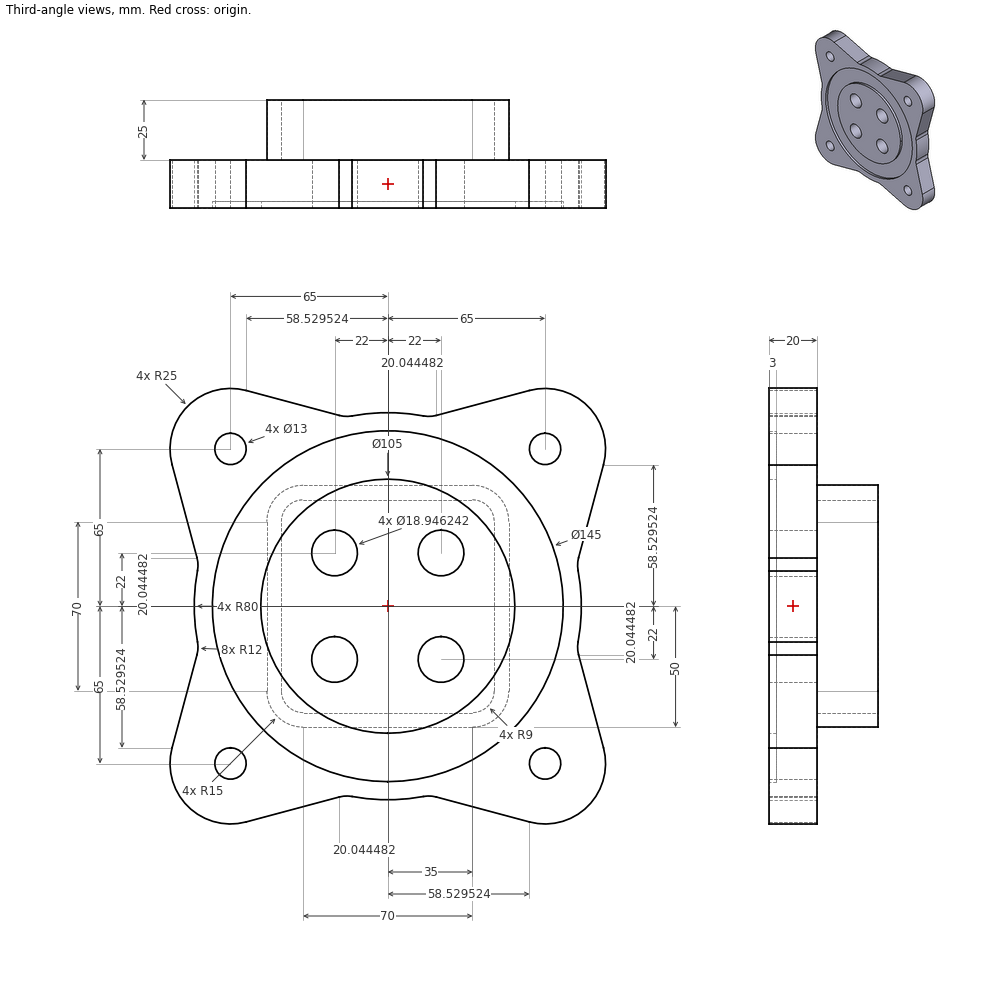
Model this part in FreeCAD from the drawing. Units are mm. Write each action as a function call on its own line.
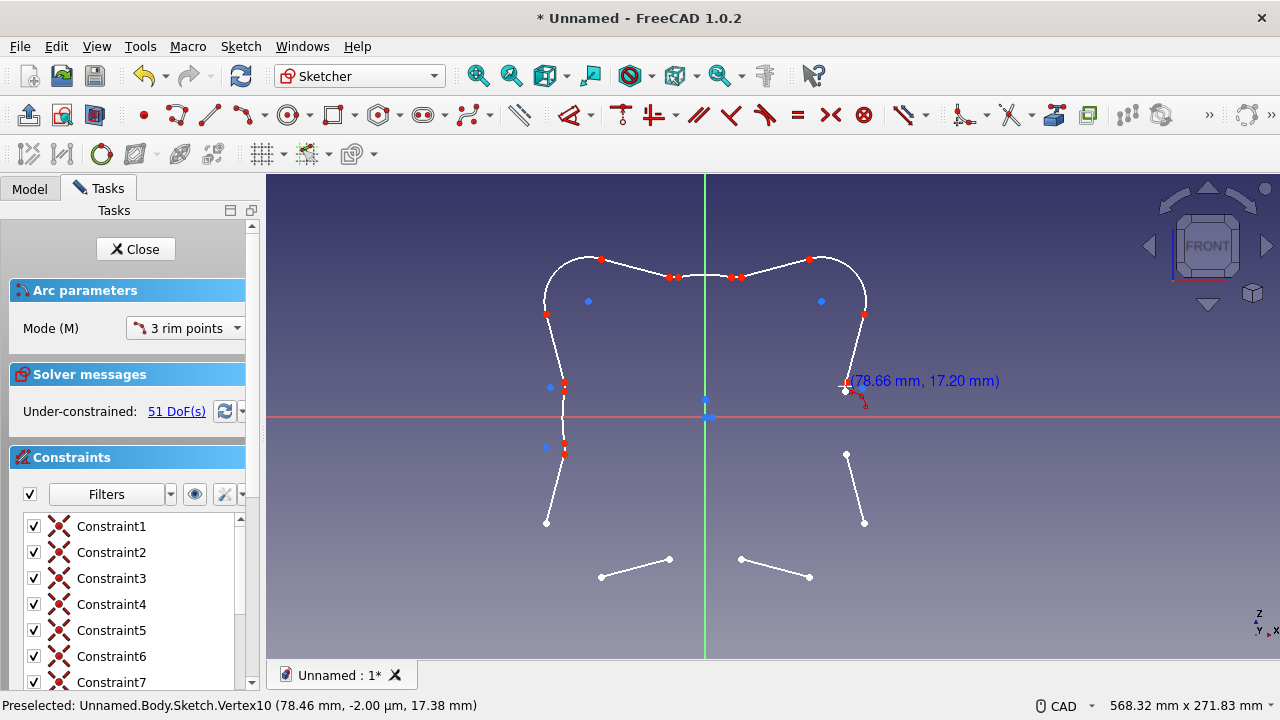
scroll(845, 391, up, 3)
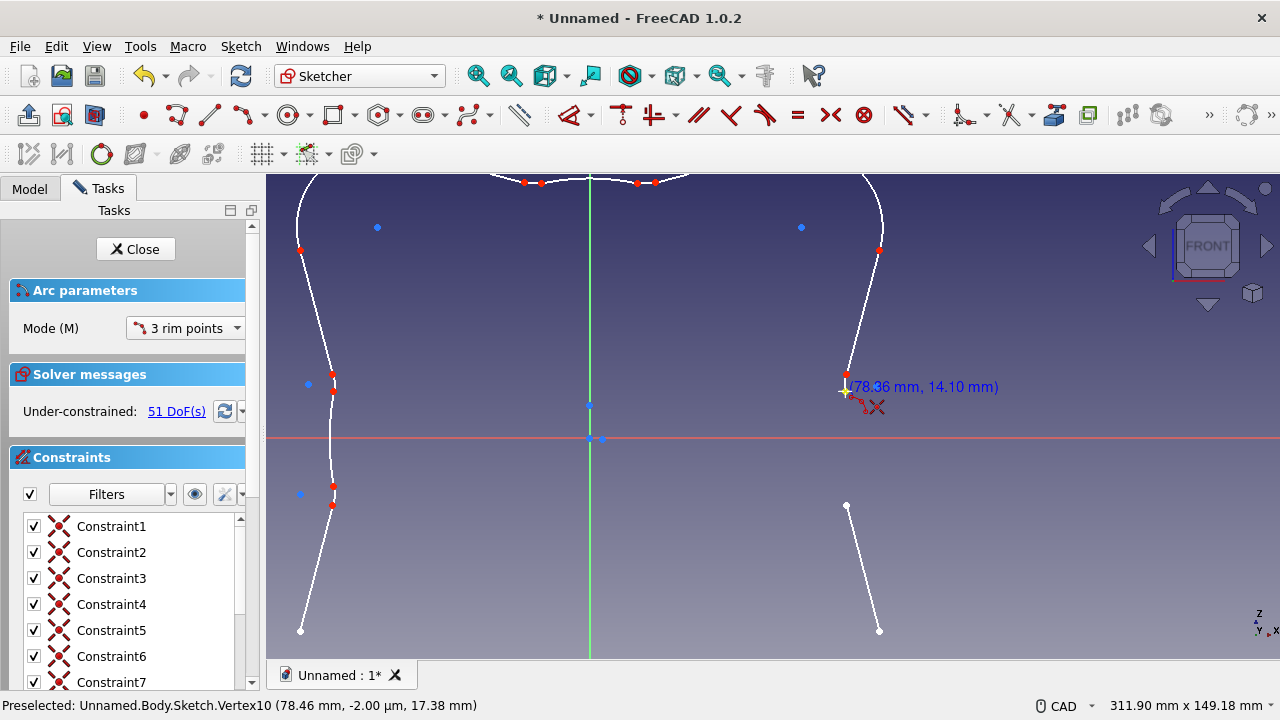
click(845, 392)
click(845, 486)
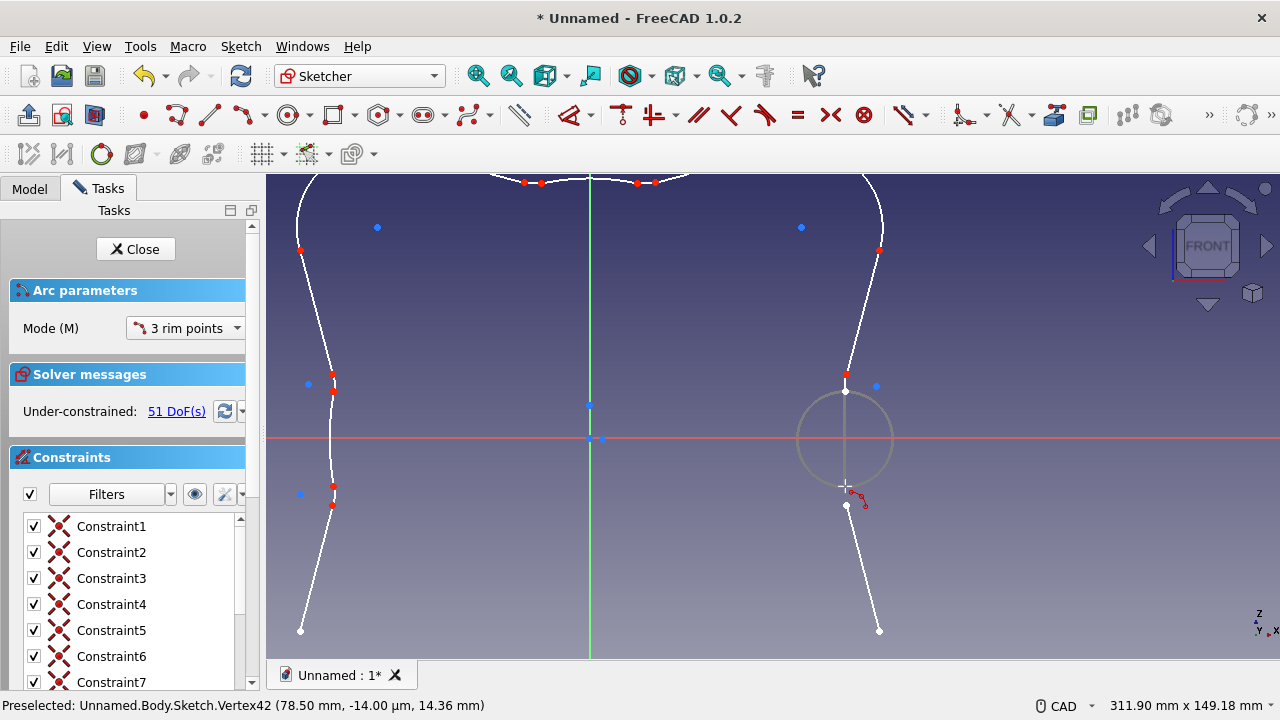
scroll(850, 448, up, 7)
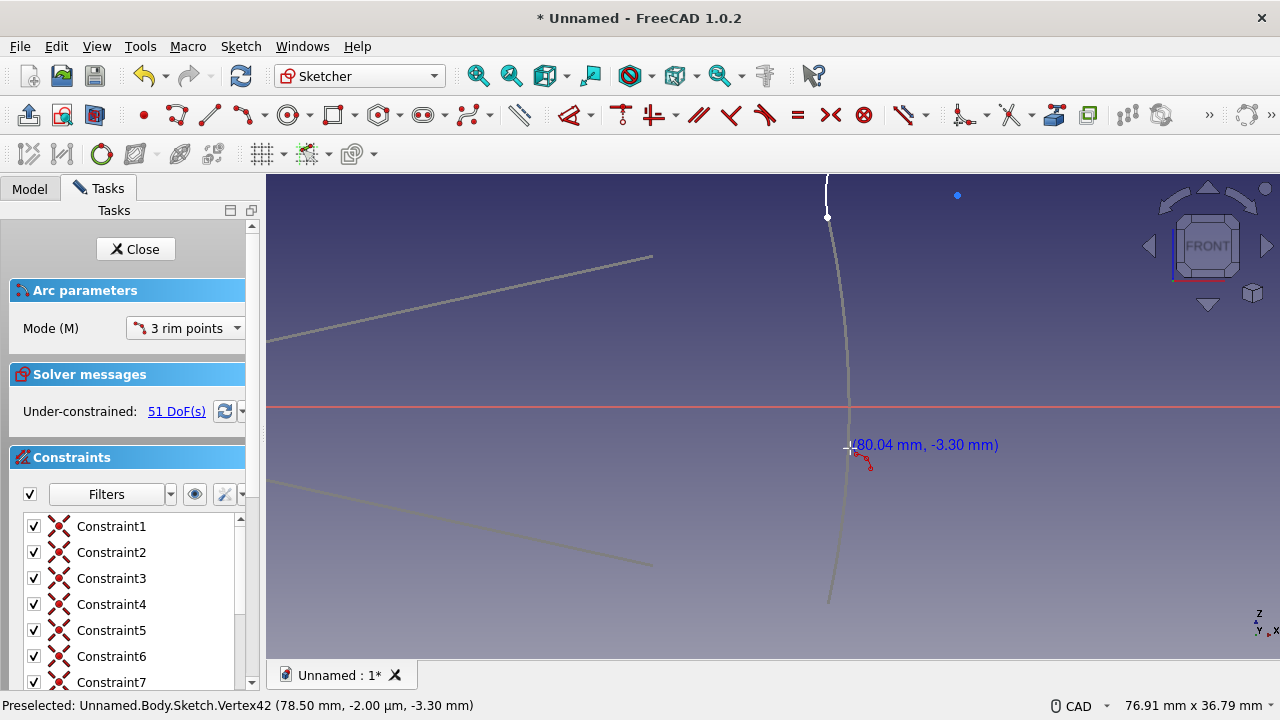
click(847, 446)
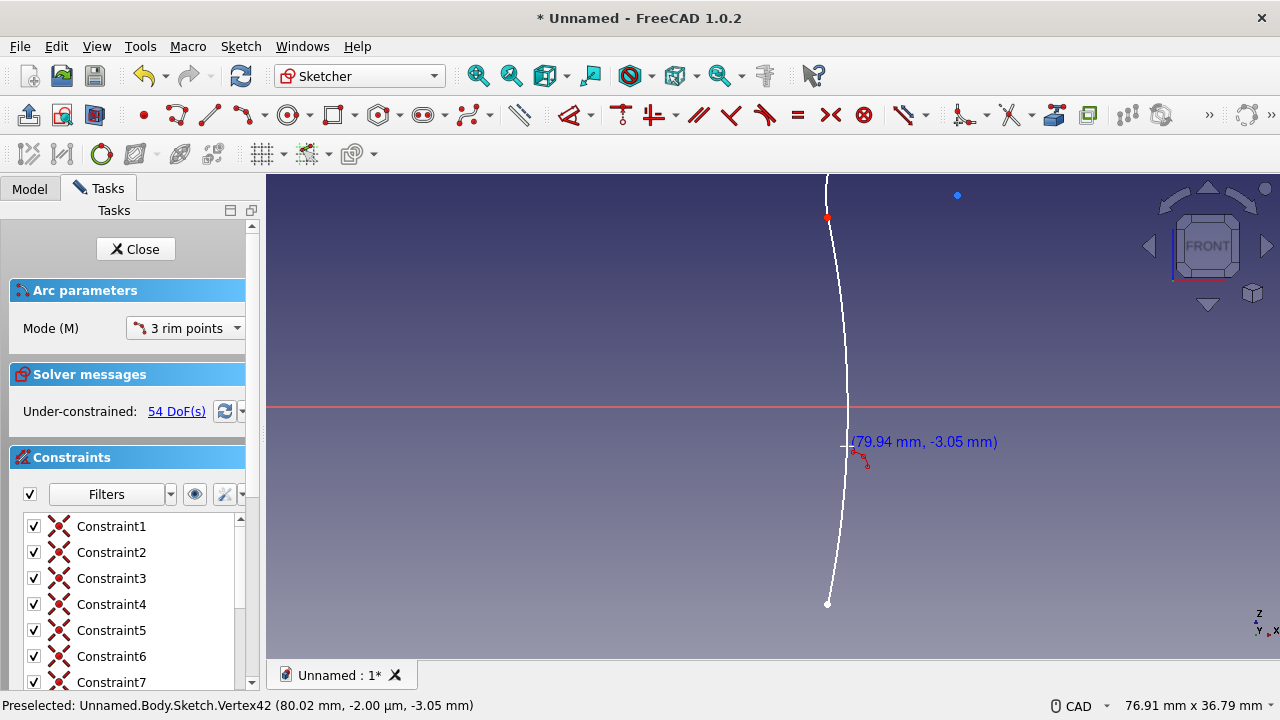
scroll(847, 418, down, 10)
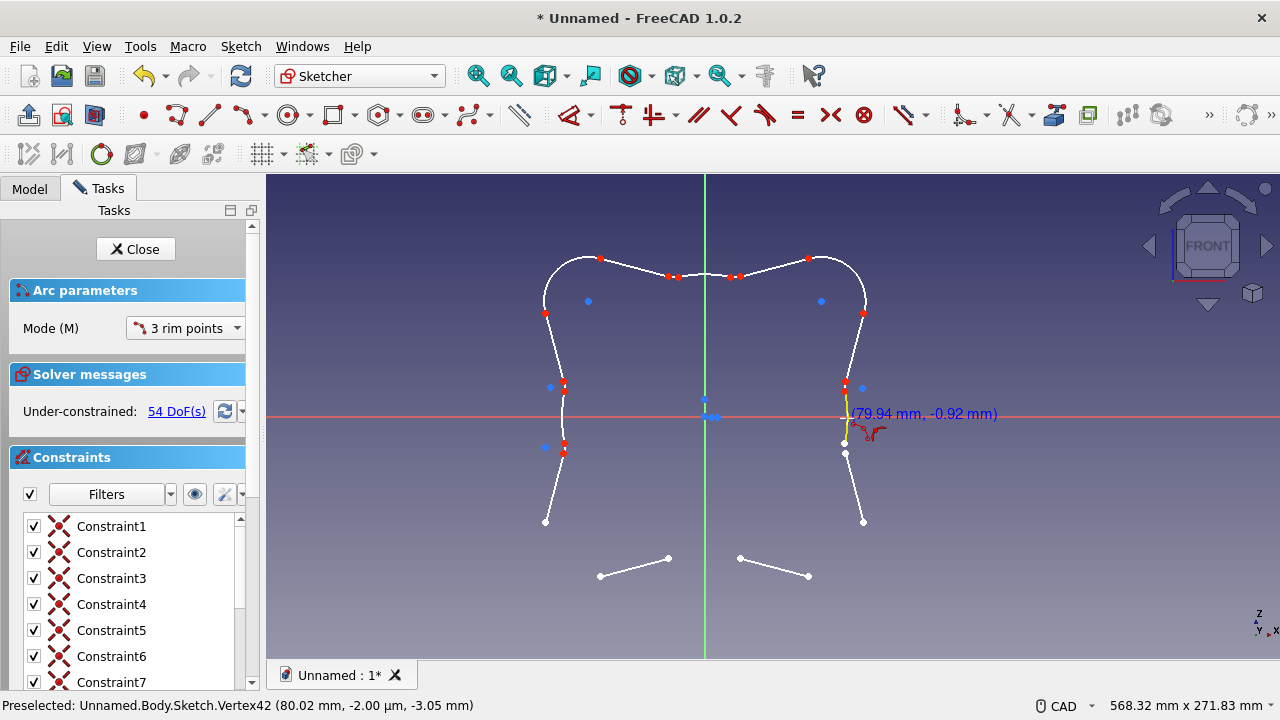
scroll(845, 443, up, 3)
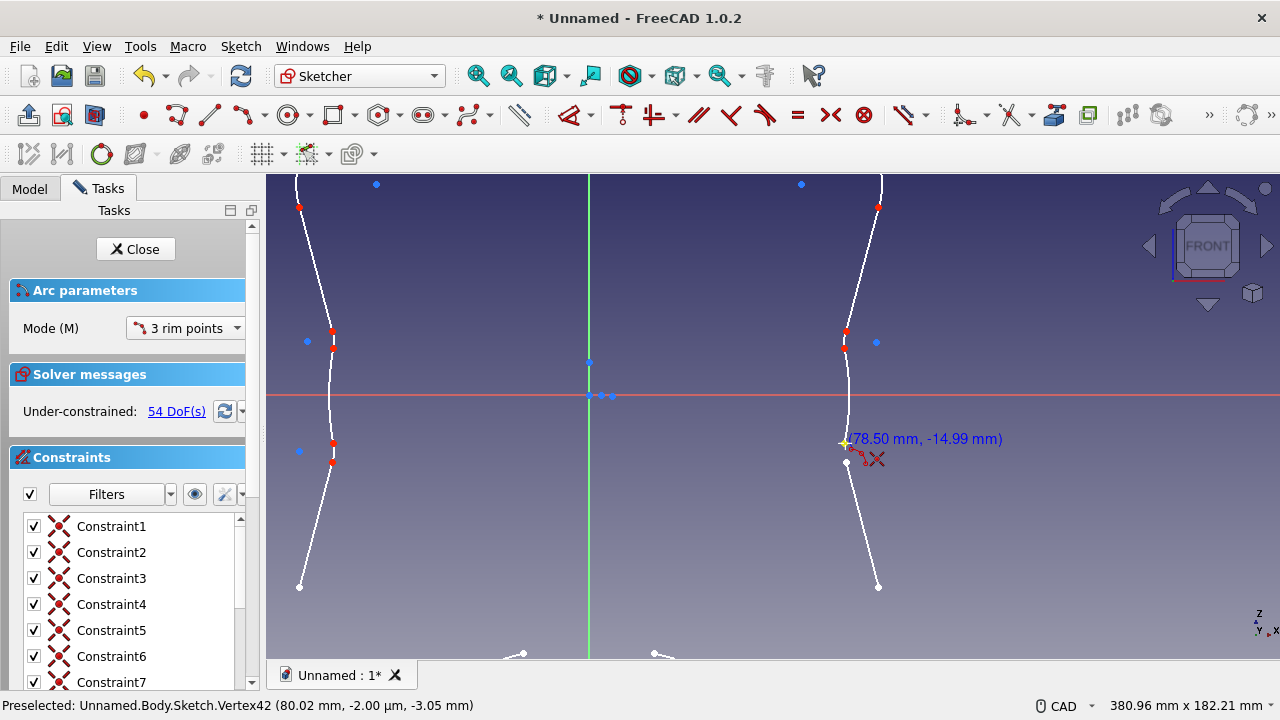
click(844, 444)
click(846, 462)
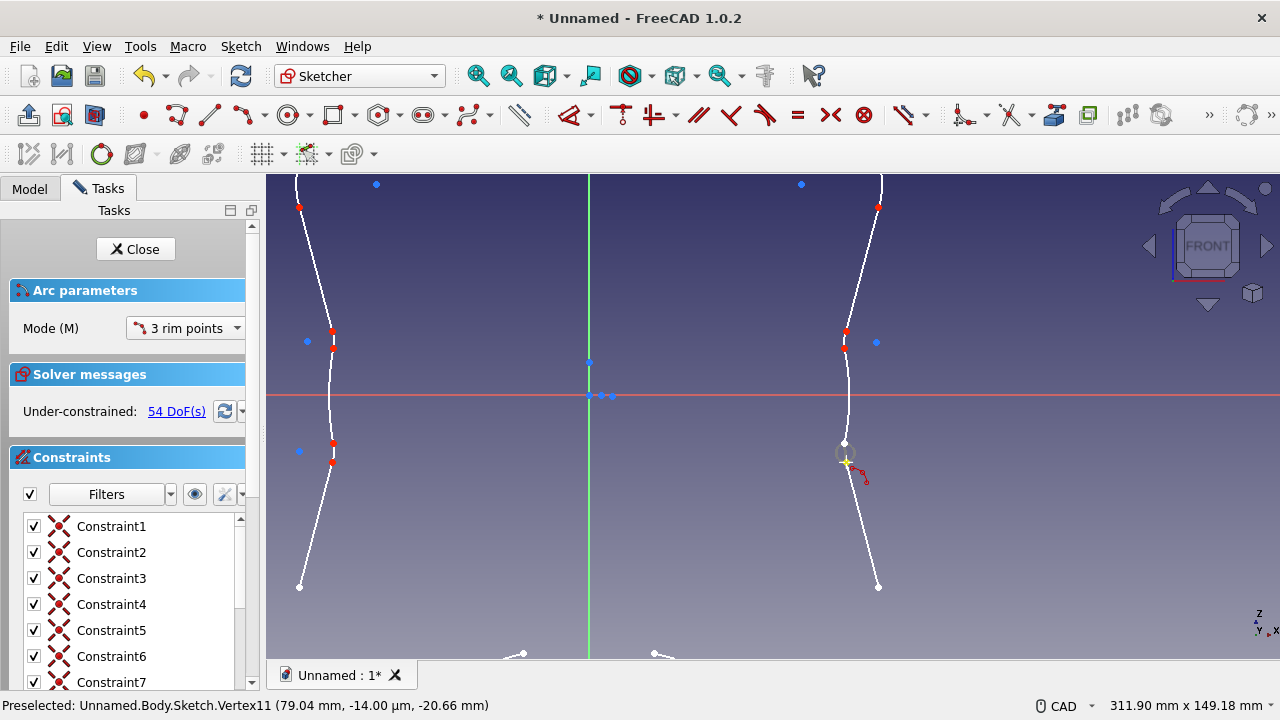
scroll(844, 452, up, 14)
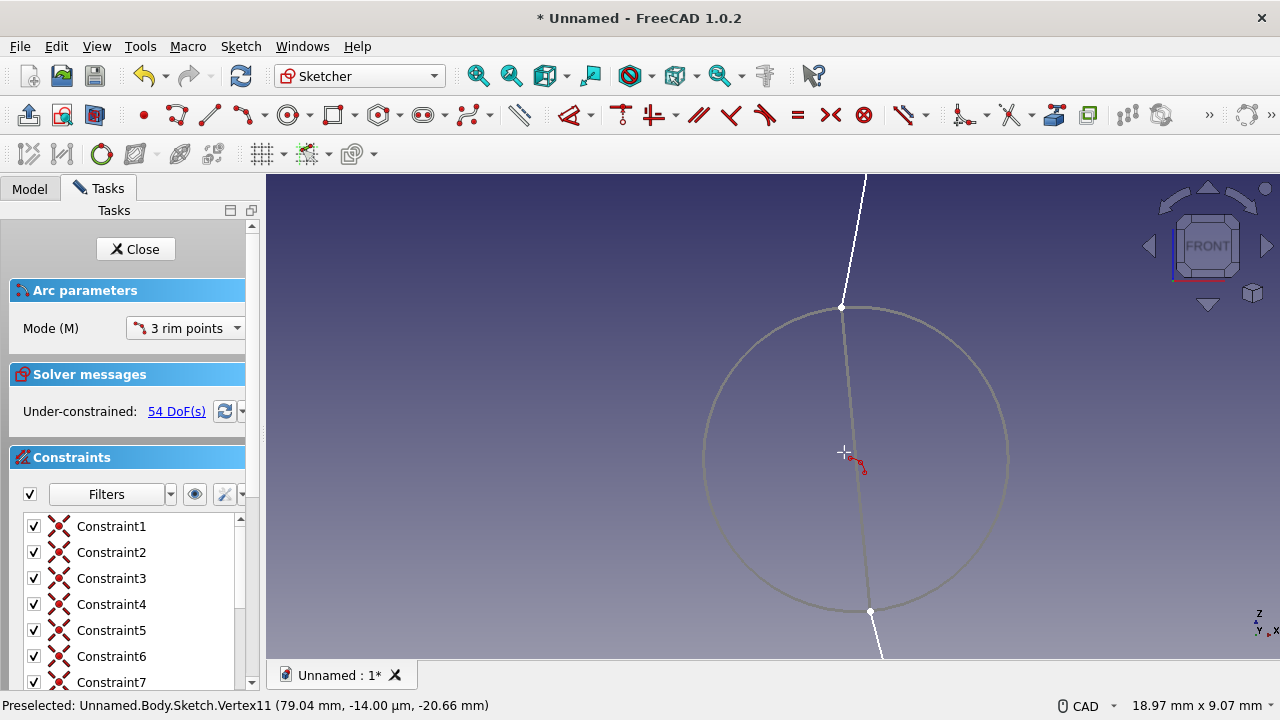
click(838, 437)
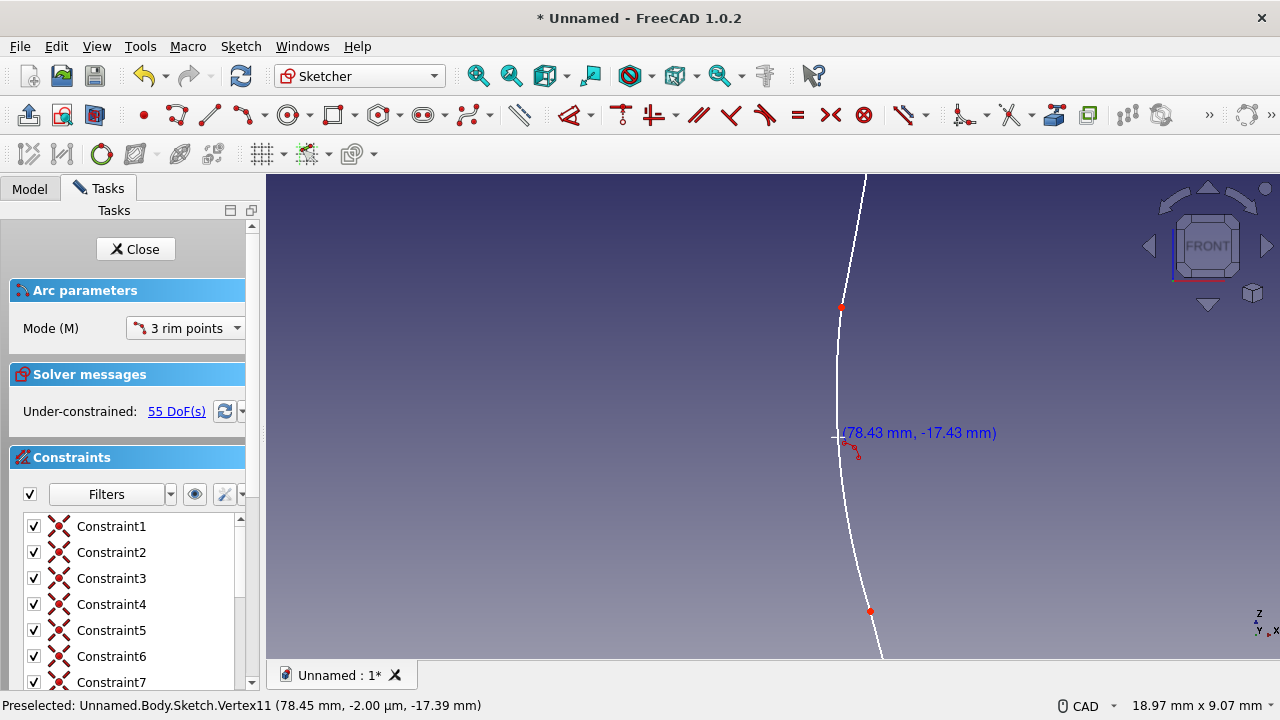
scroll(845, 448, down, 17)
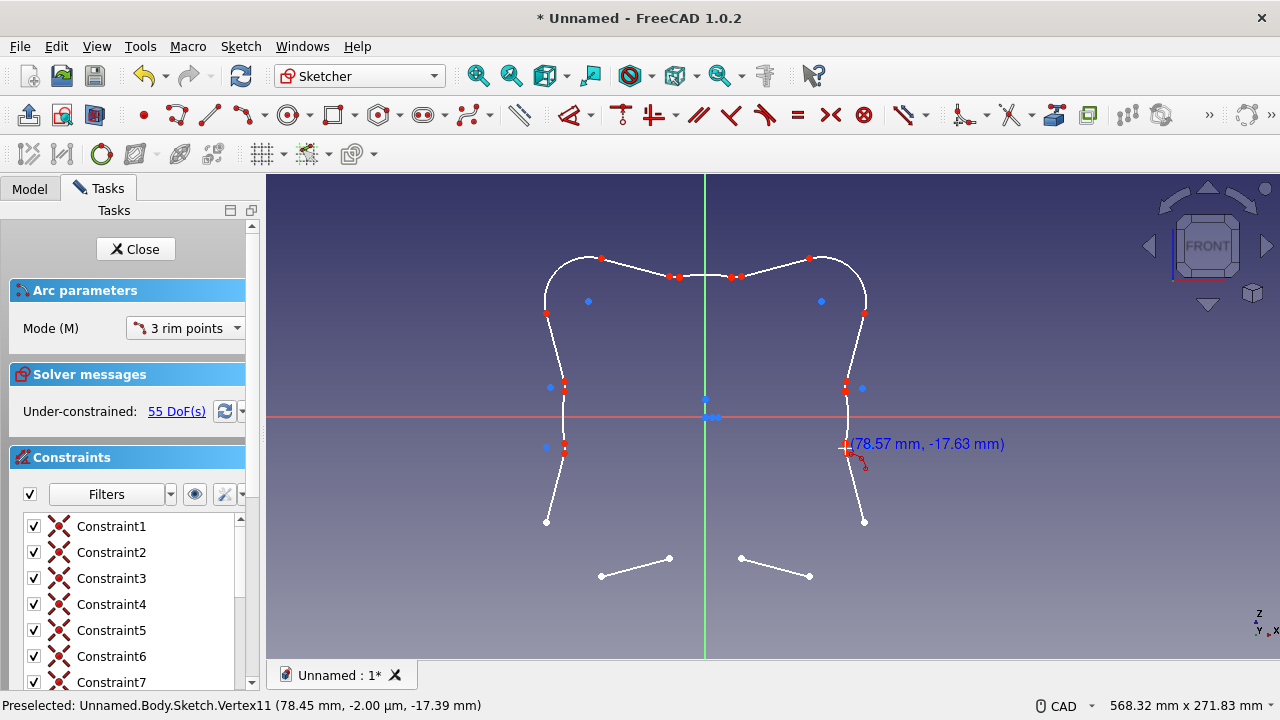
click(864, 523)
click(809, 577)
click(853, 565)